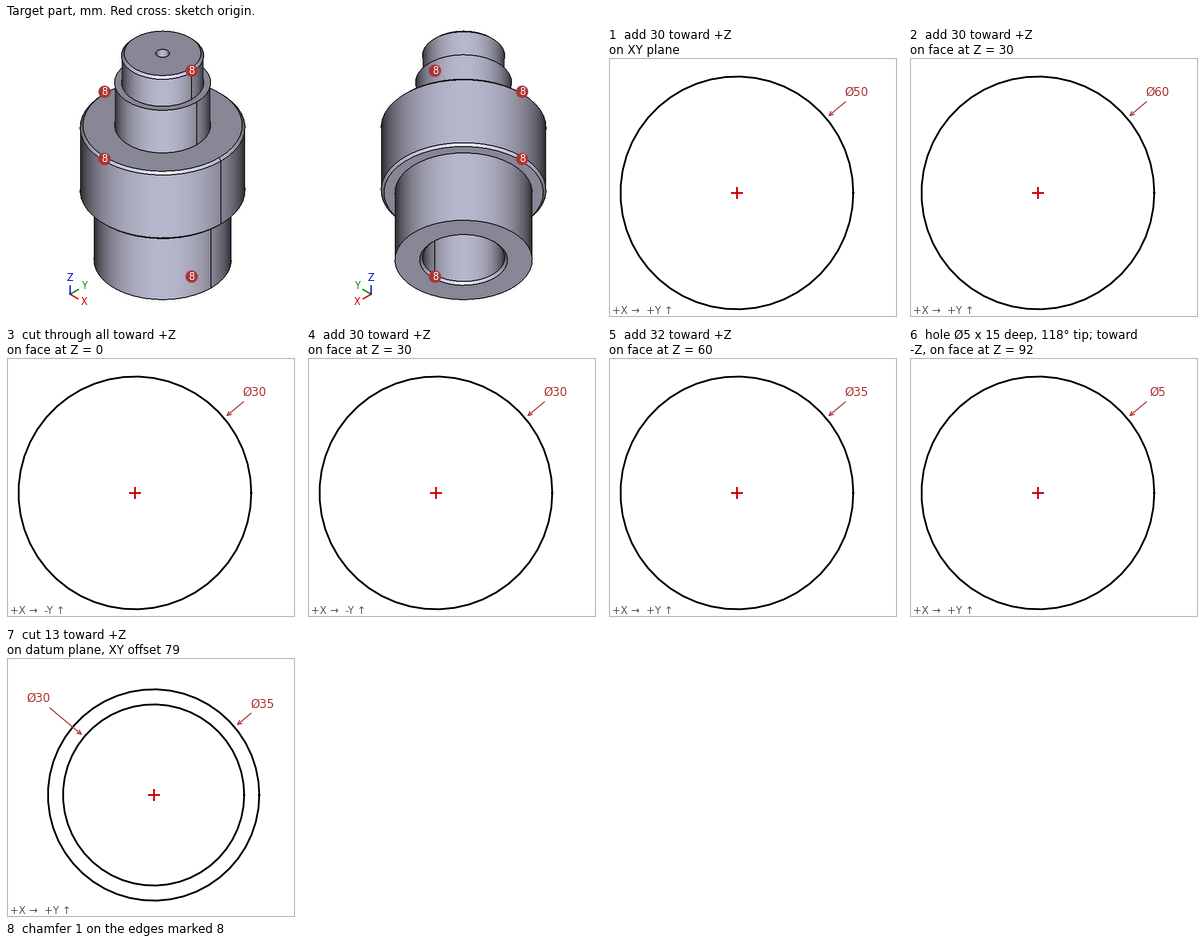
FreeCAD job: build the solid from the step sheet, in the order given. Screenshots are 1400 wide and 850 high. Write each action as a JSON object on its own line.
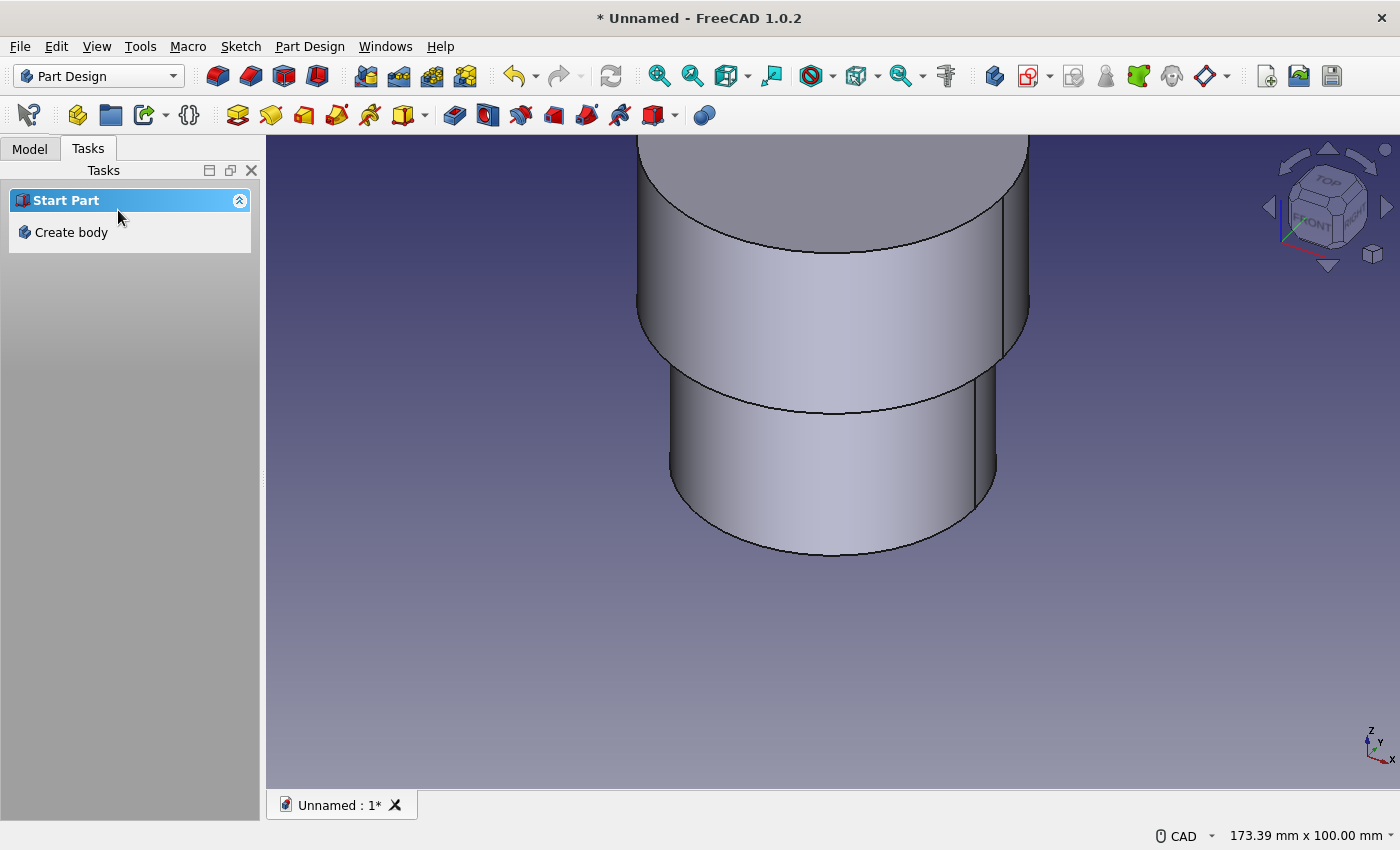
{"action": "key", "text": "v f"}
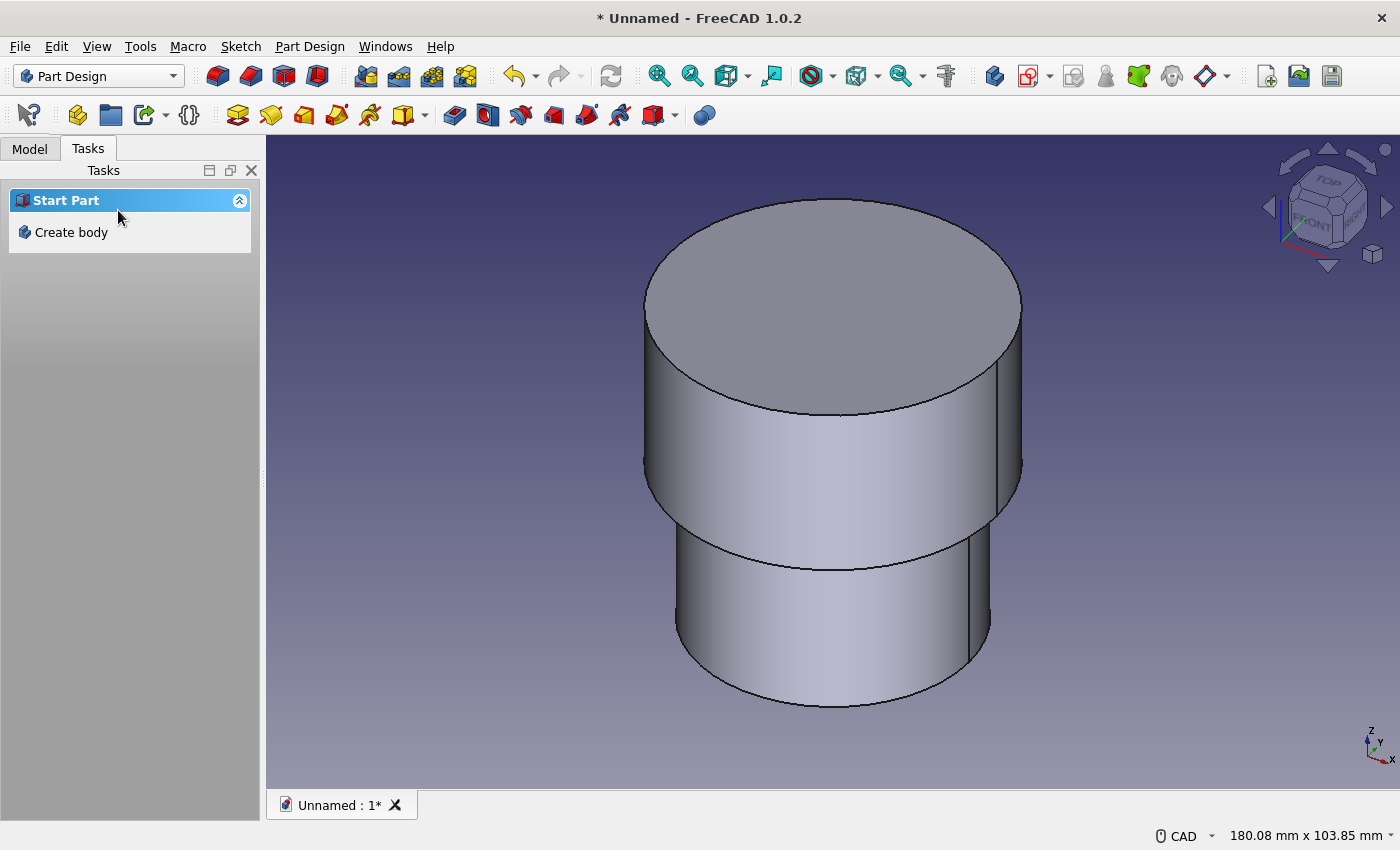
{"action": "key", "text": "5"}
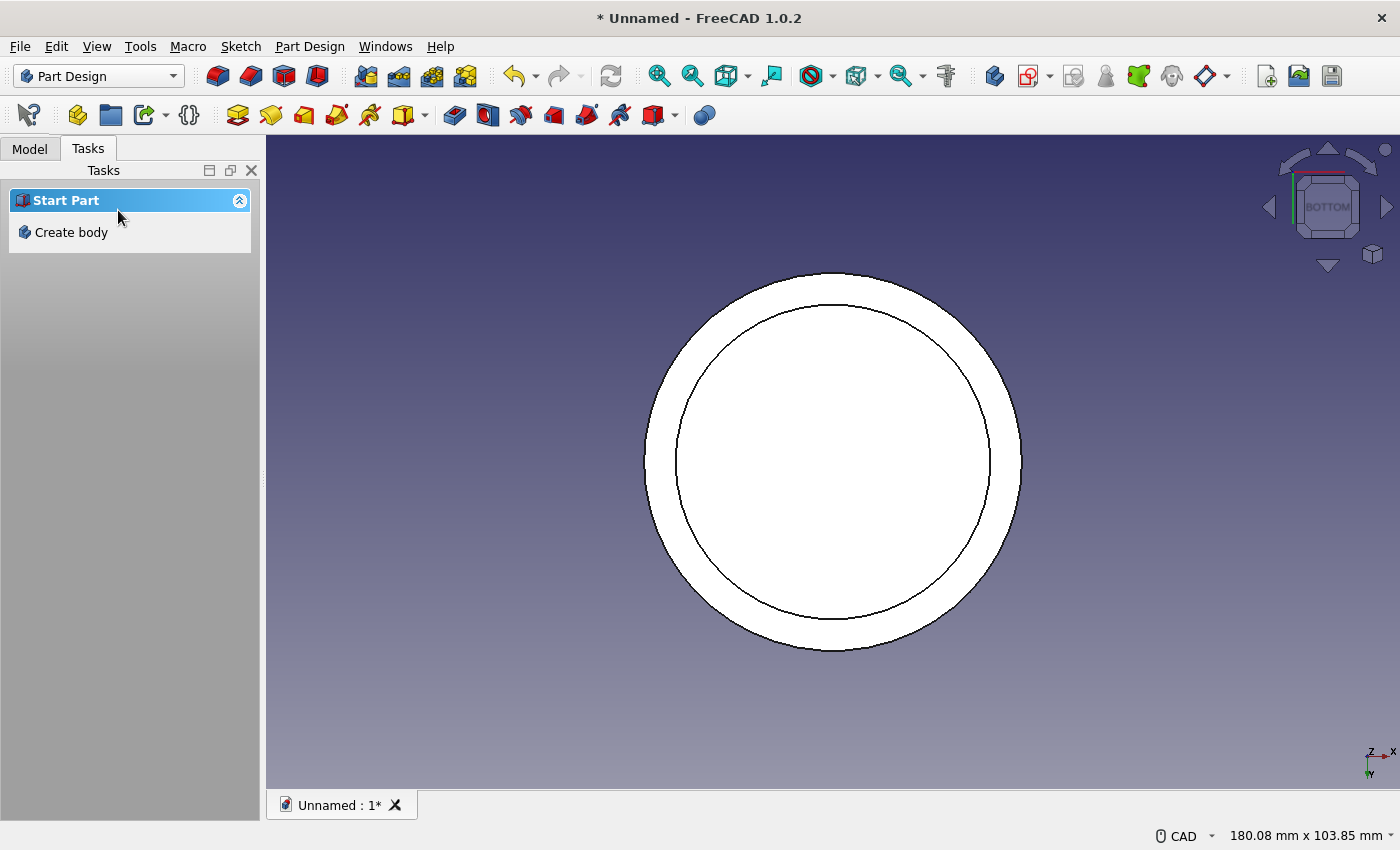
{"action": "left_click", "coordinate": [833, 461]}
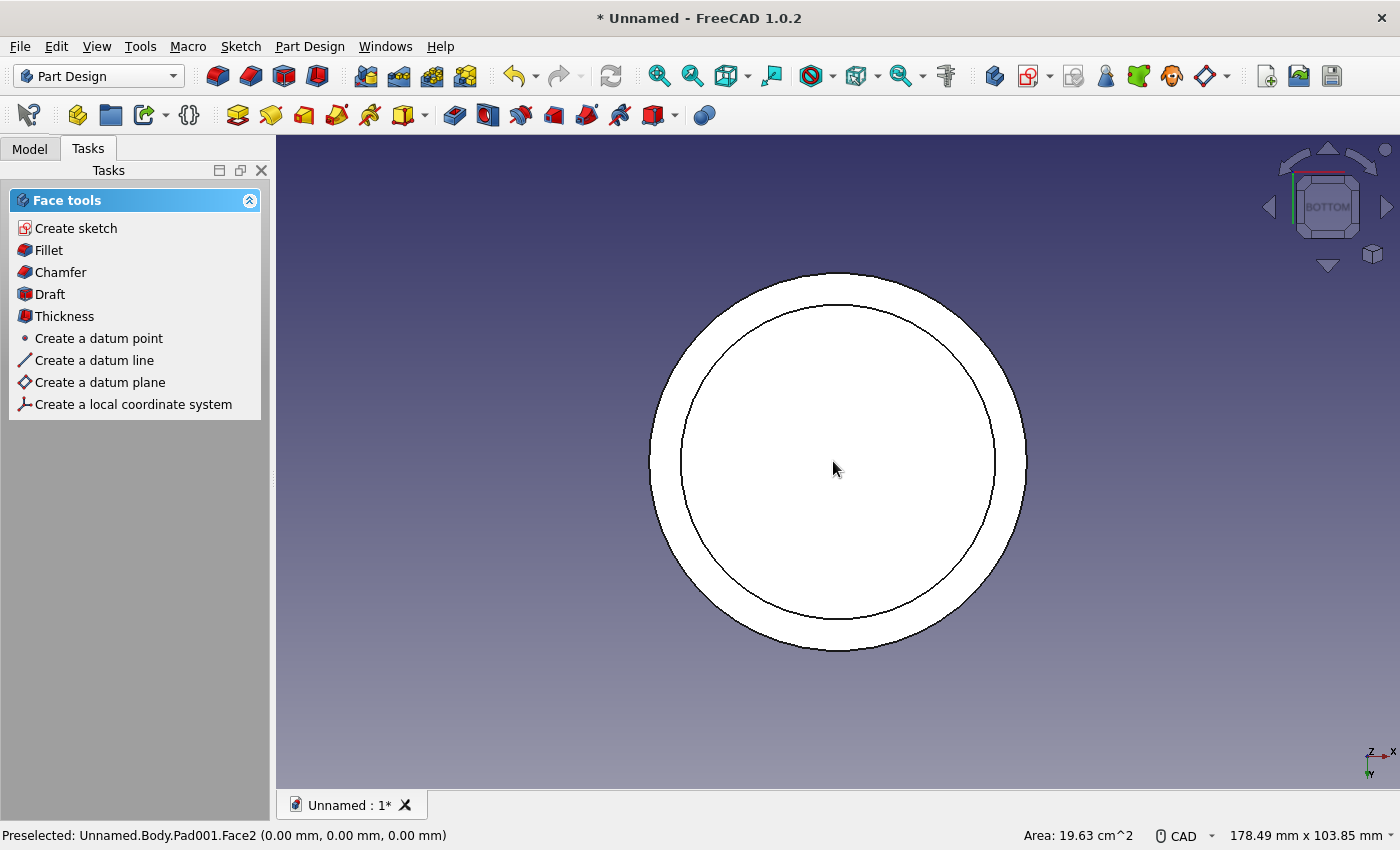
{"action": "left_click", "coordinate": [1028, 76]}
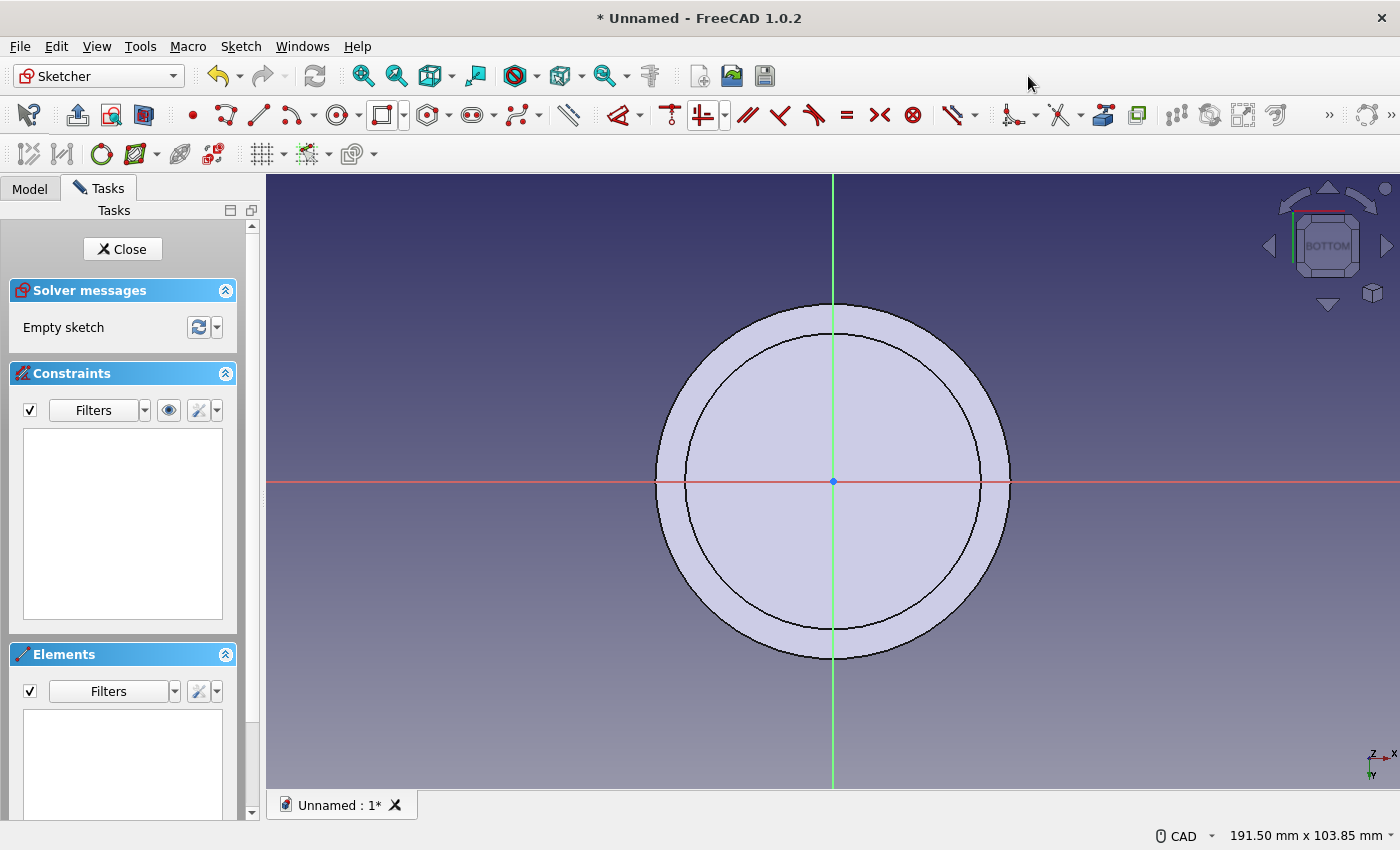
{"action": "scroll", "coordinate": [889, 482], "scroll_direction": "up", "scroll_amount": 4}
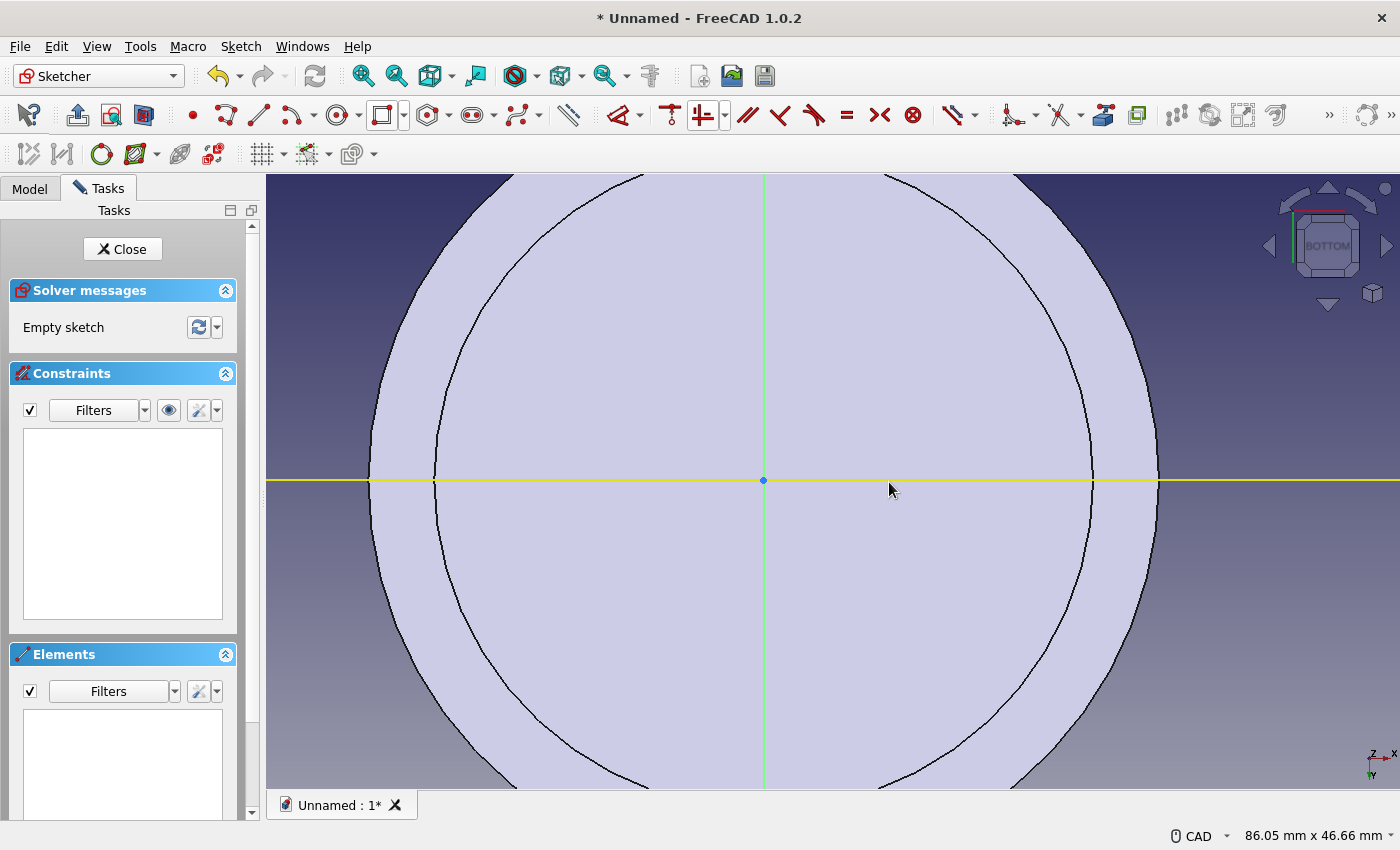
{"action": "key", "text": "g c"}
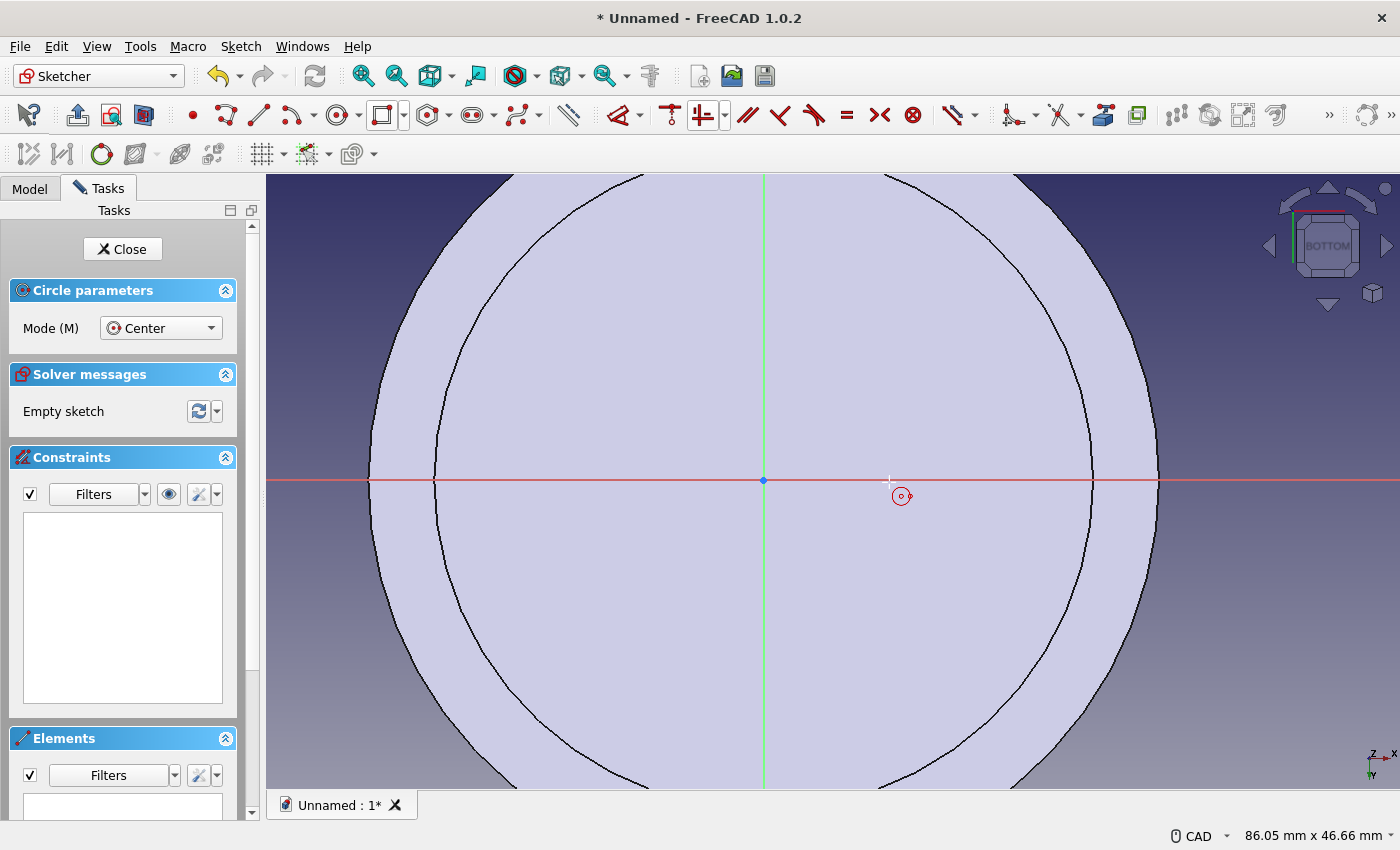
{"action": "left_click", "coordinate": [764, 480]}
{"action": "left_click", "coordinate": [903, 340]}
{"action": "key", "text": "Escape"}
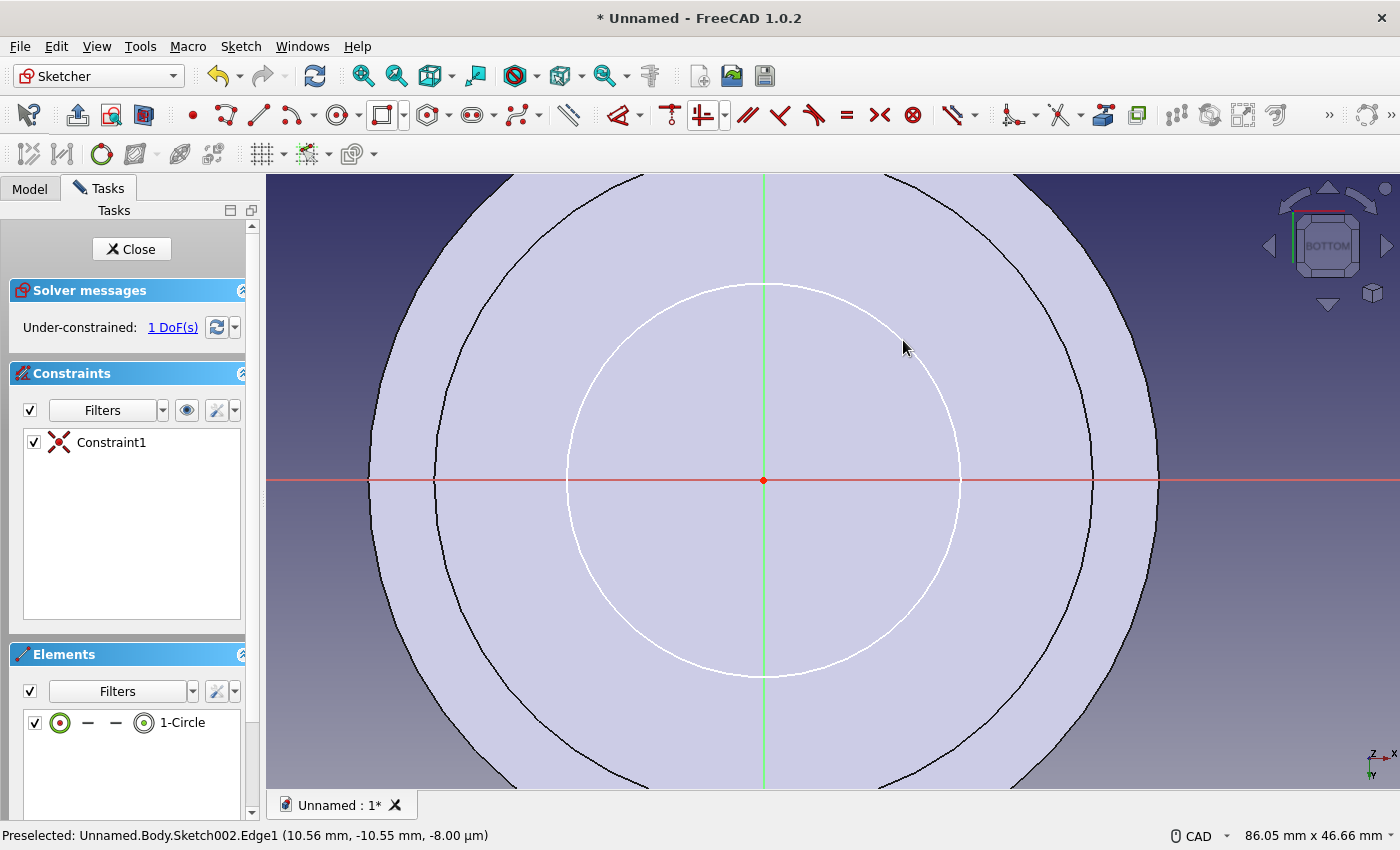
{"action": "key", "text": "d"}